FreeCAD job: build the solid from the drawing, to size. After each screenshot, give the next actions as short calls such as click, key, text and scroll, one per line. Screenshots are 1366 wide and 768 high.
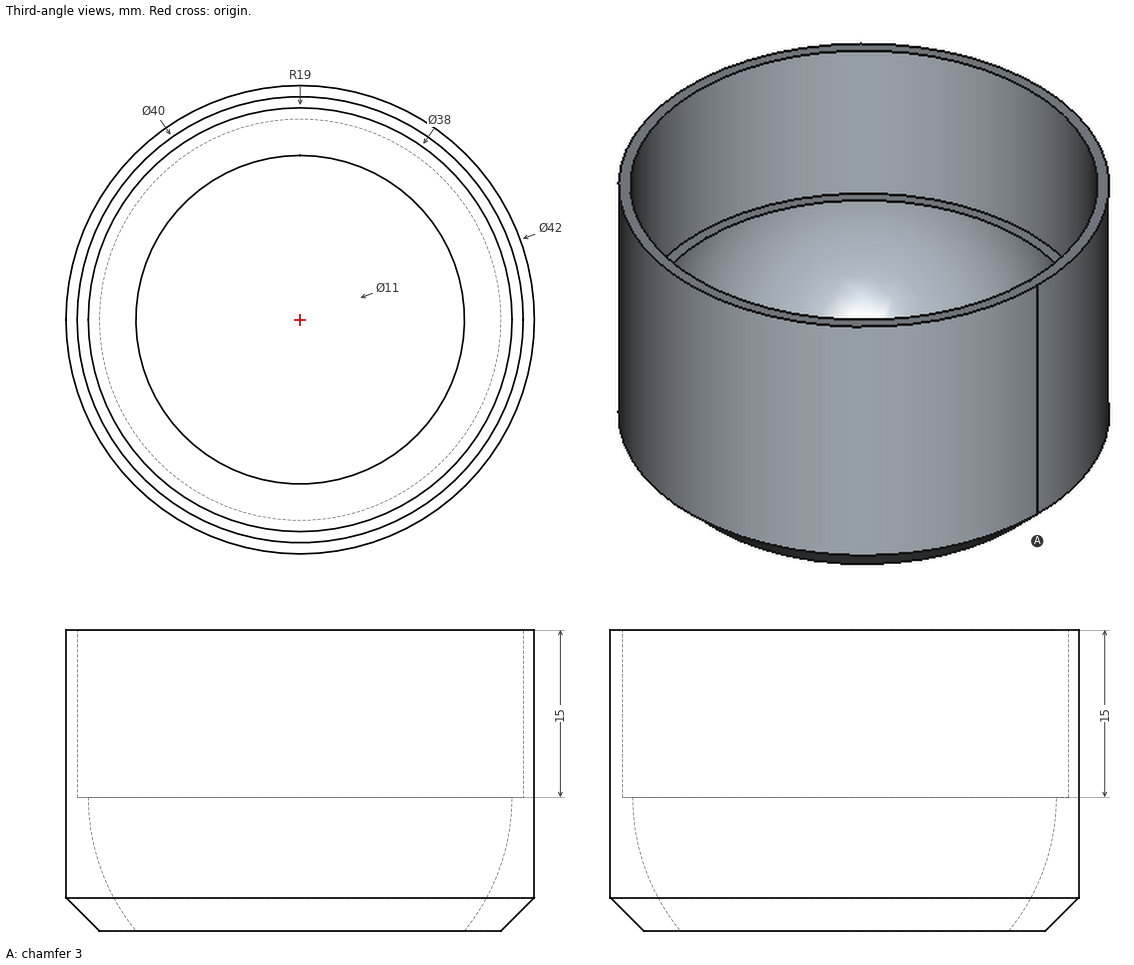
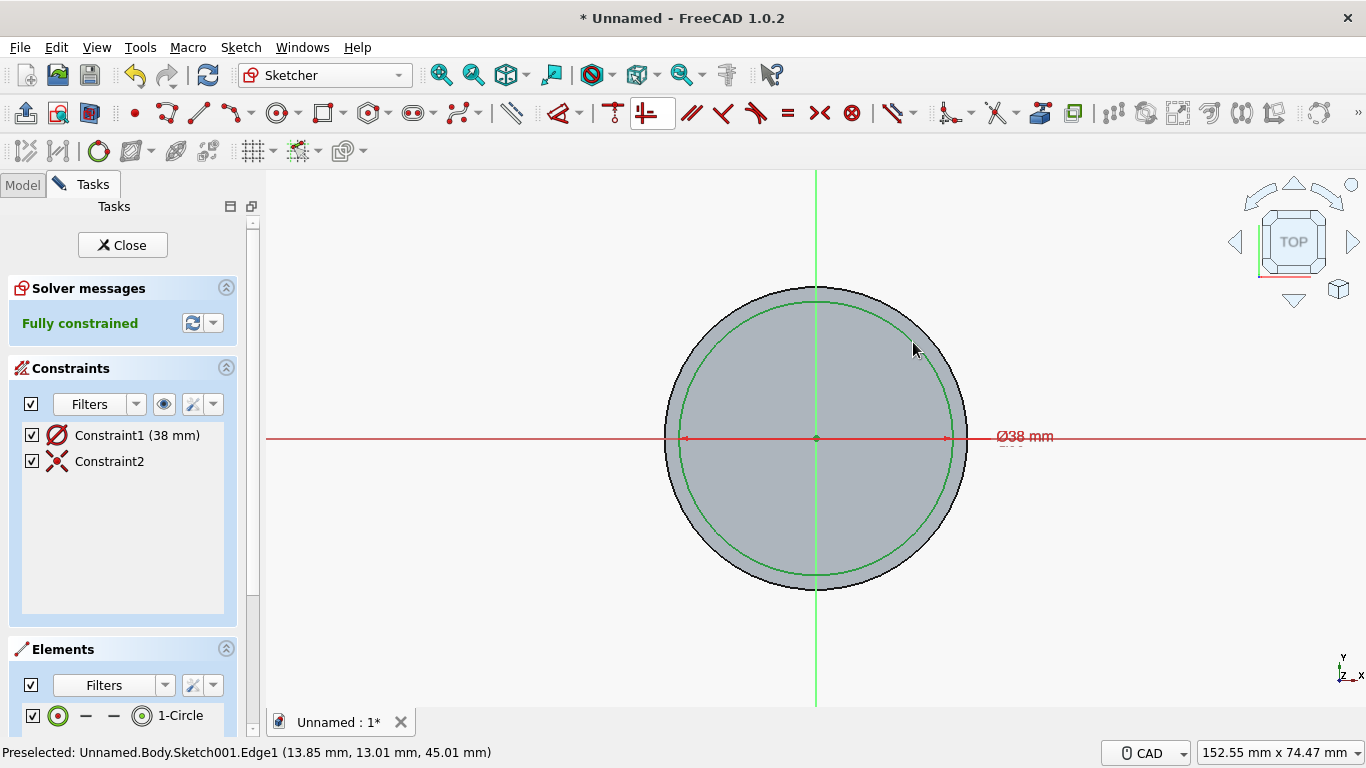
click(123, 245)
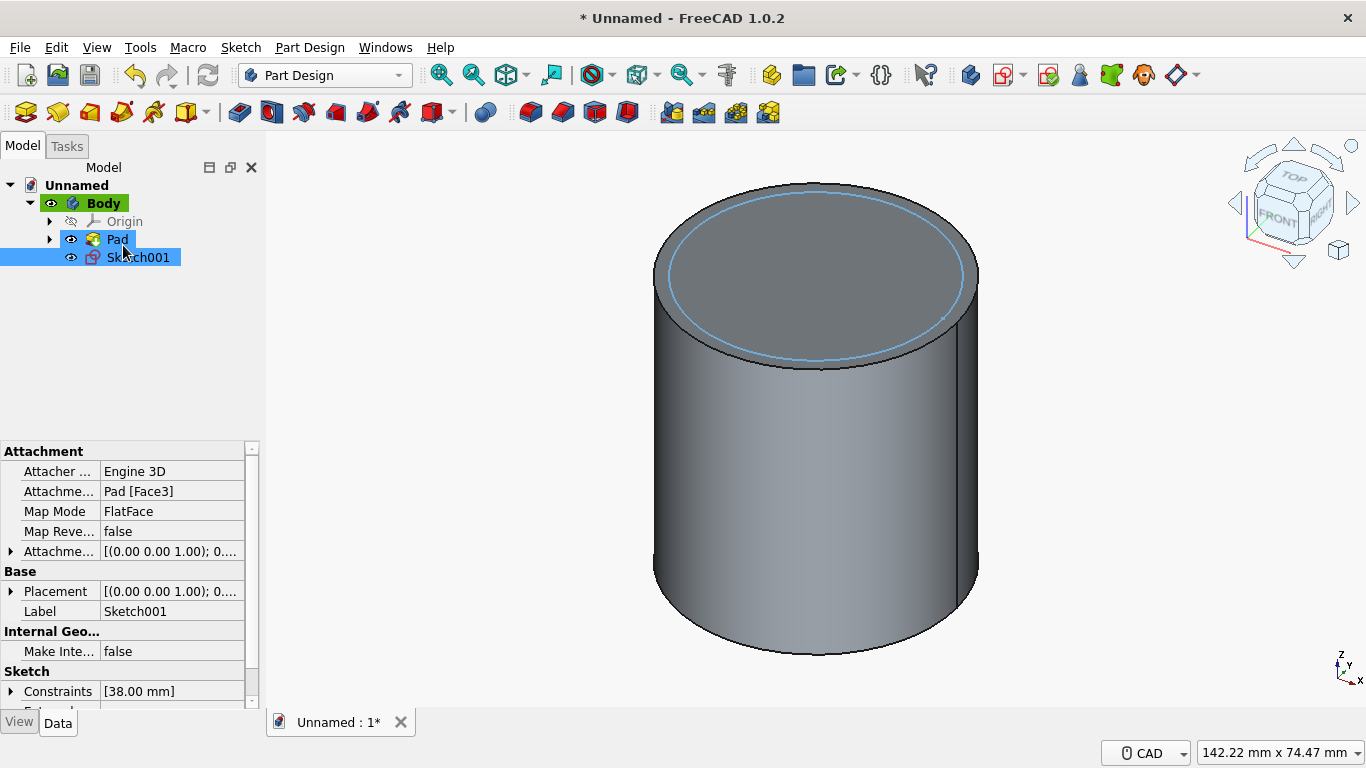
click(240, 112)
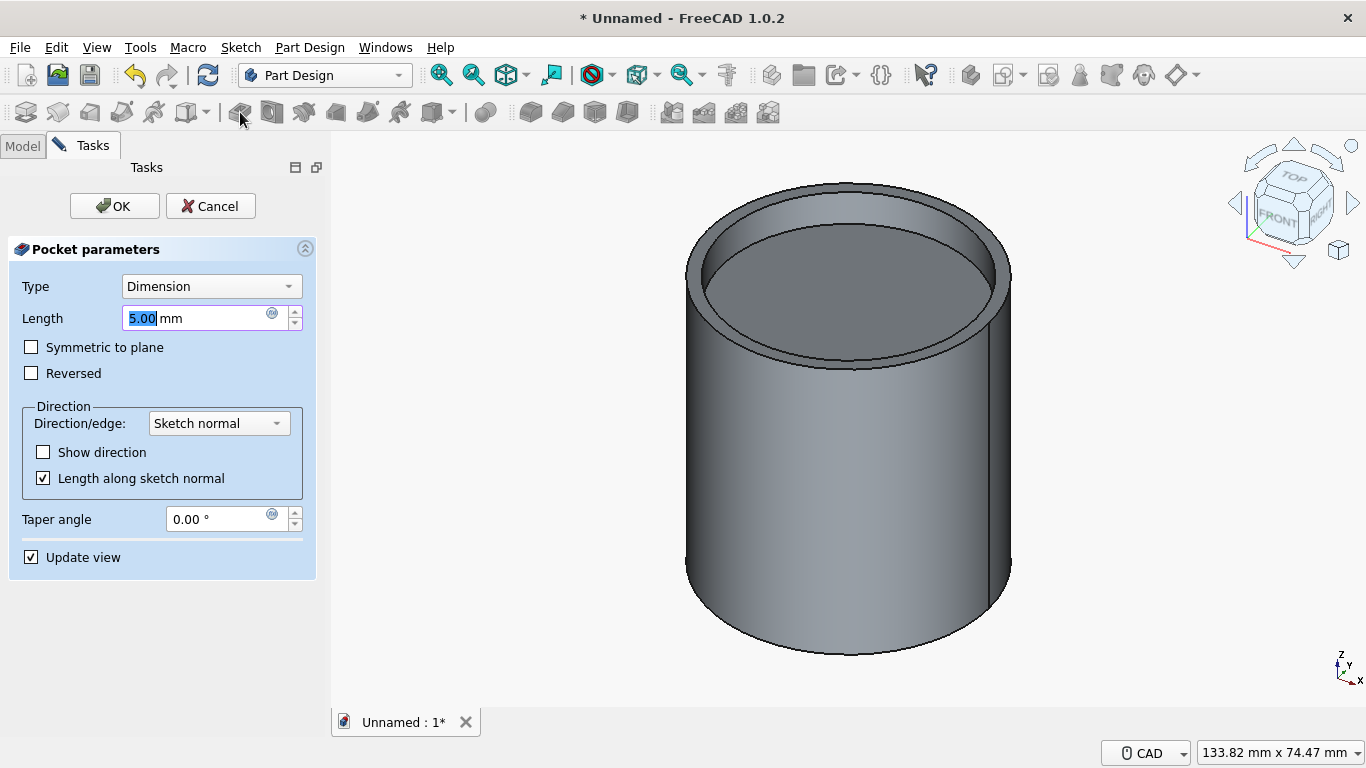
text(15)
key(Tab)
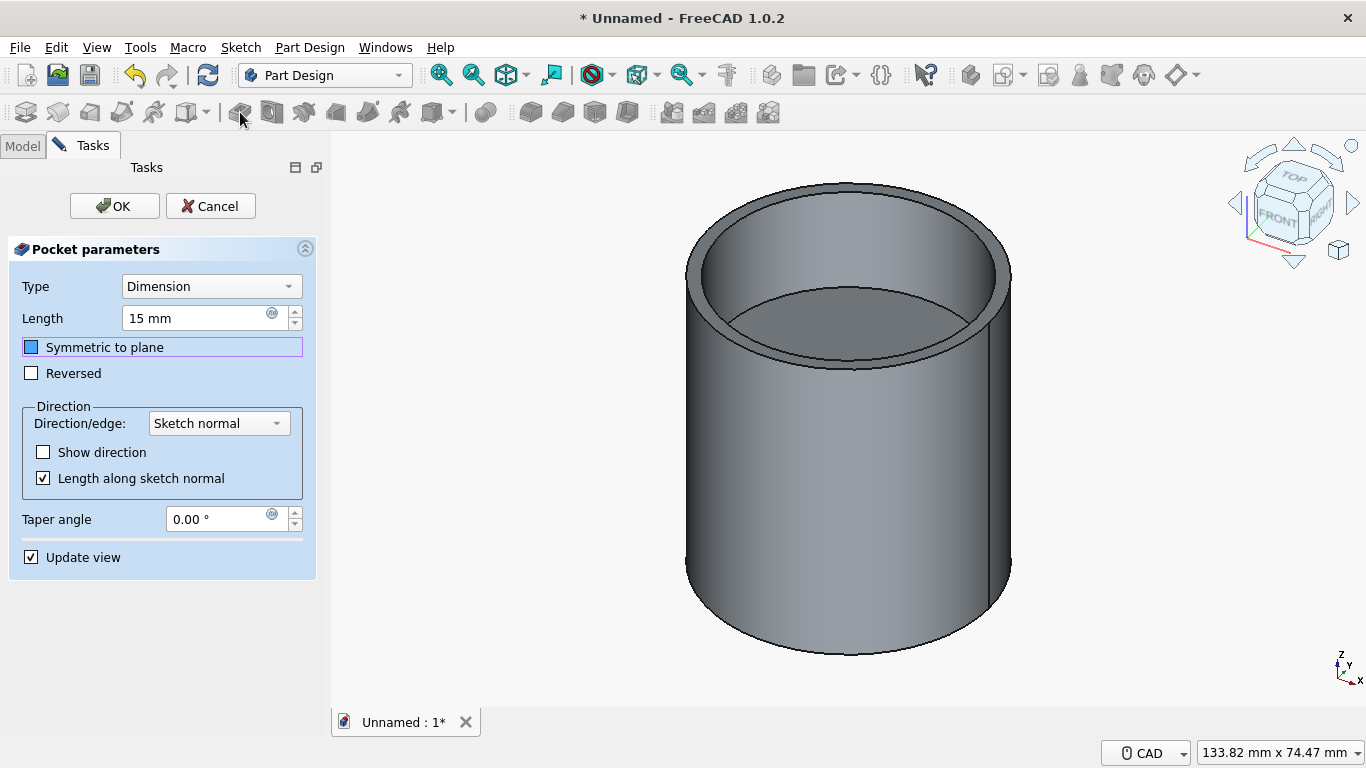
click(115, 206)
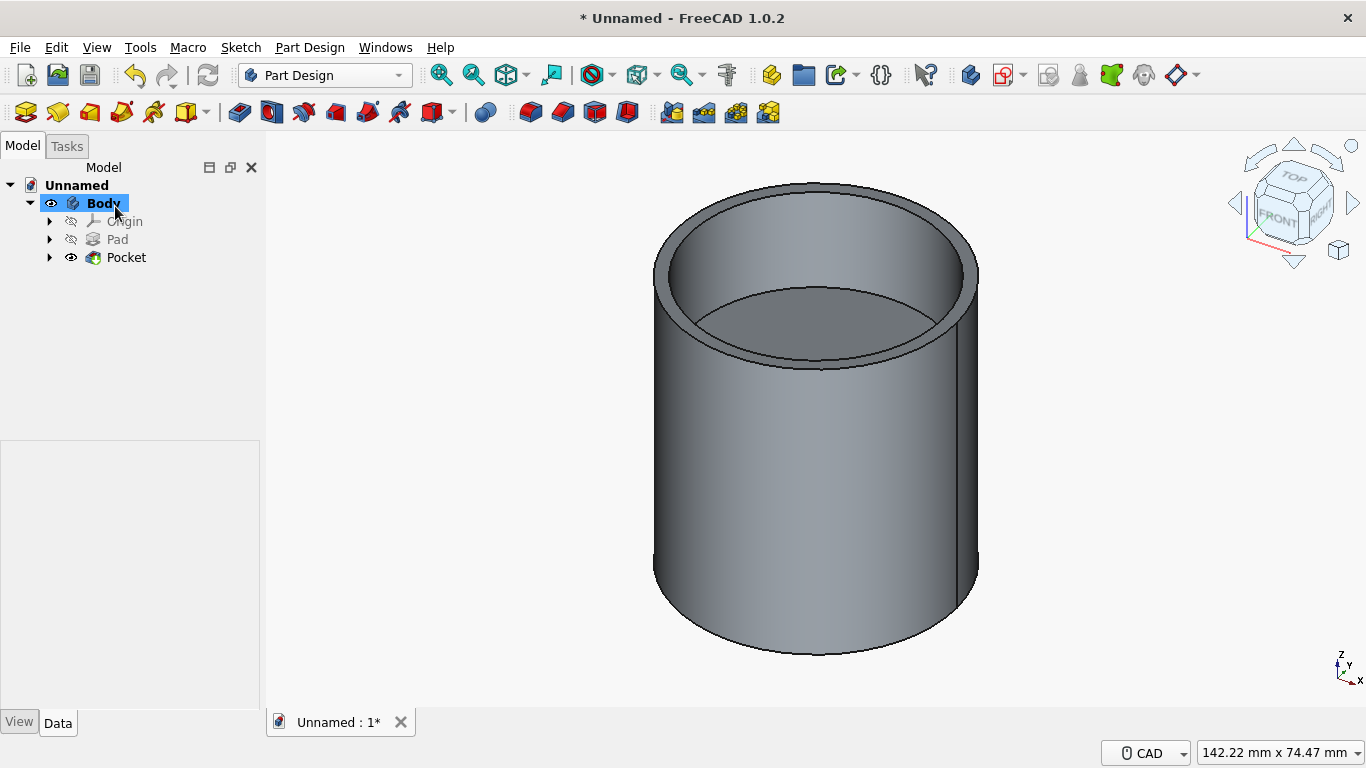
click(837, 350)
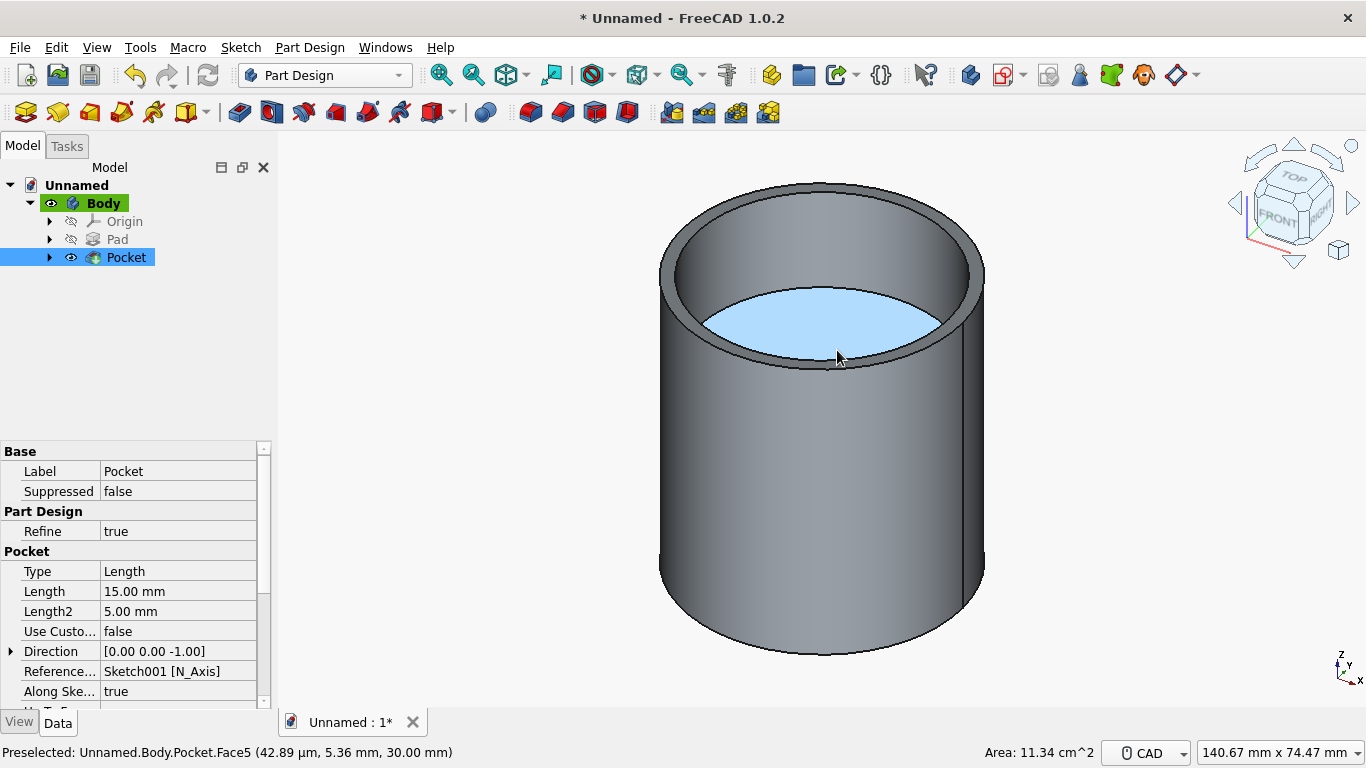
click(1004, 76)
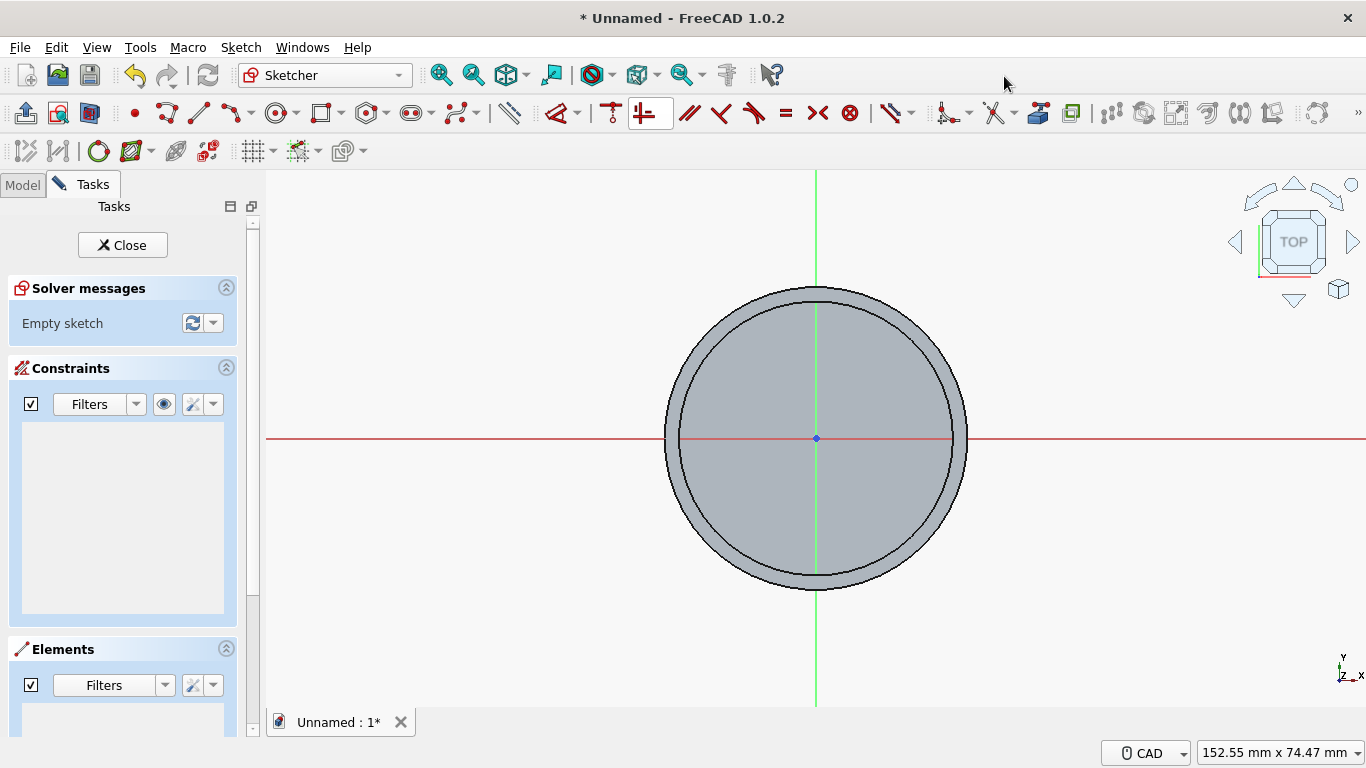
click(90, 114)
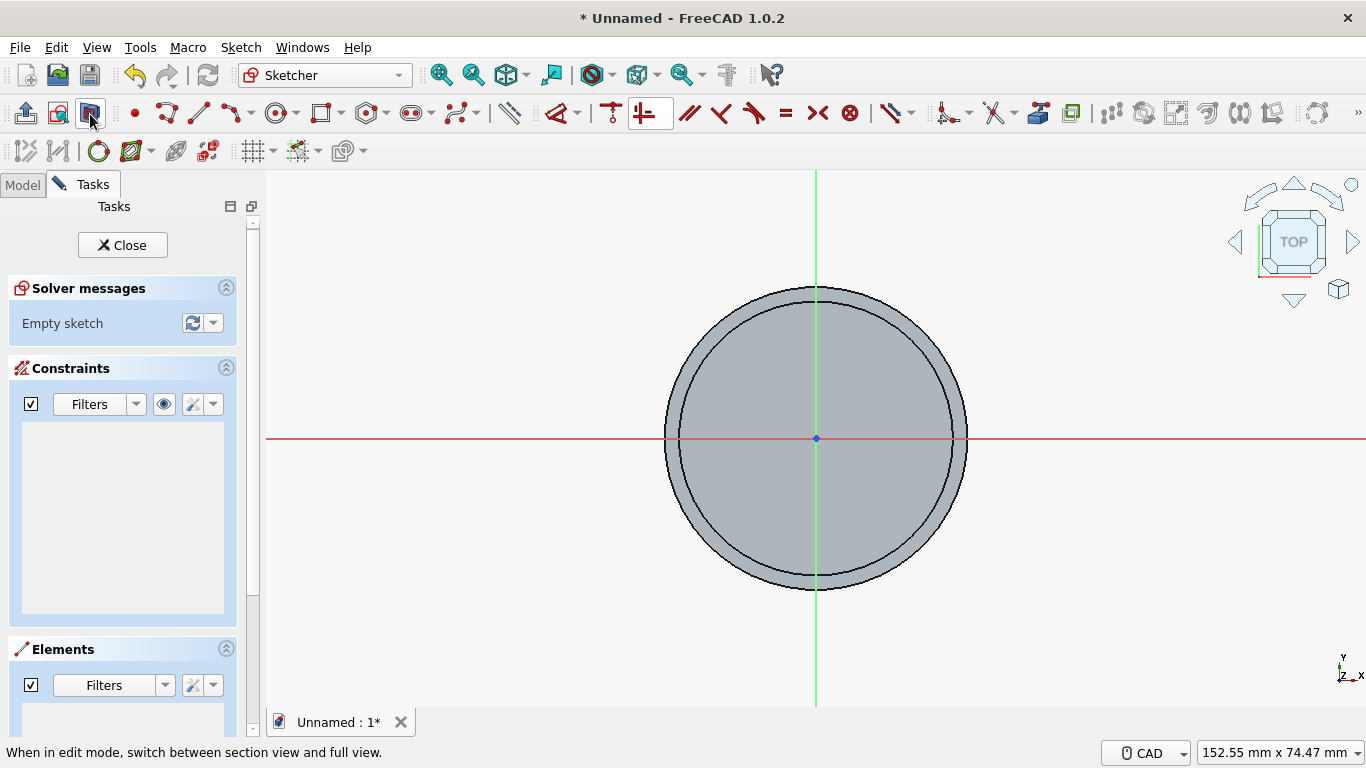
scroll(872, 314, up, 4)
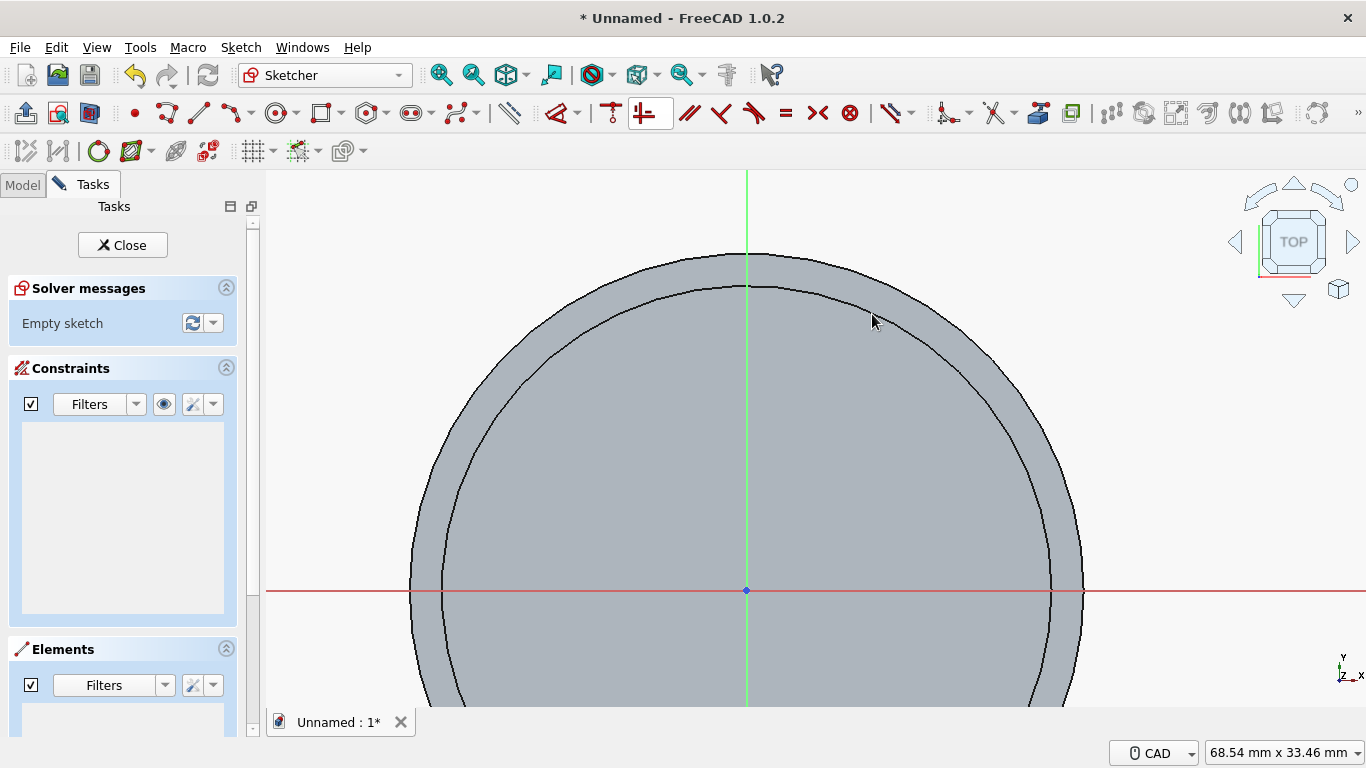
click(200, 114)